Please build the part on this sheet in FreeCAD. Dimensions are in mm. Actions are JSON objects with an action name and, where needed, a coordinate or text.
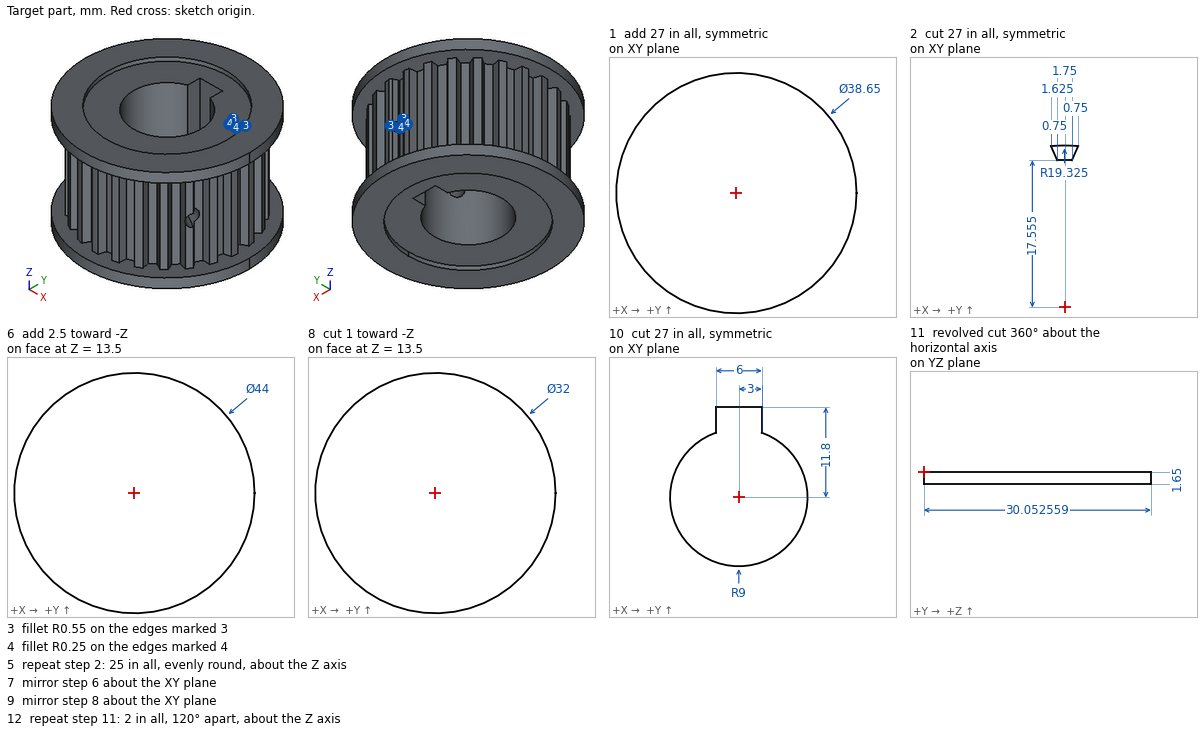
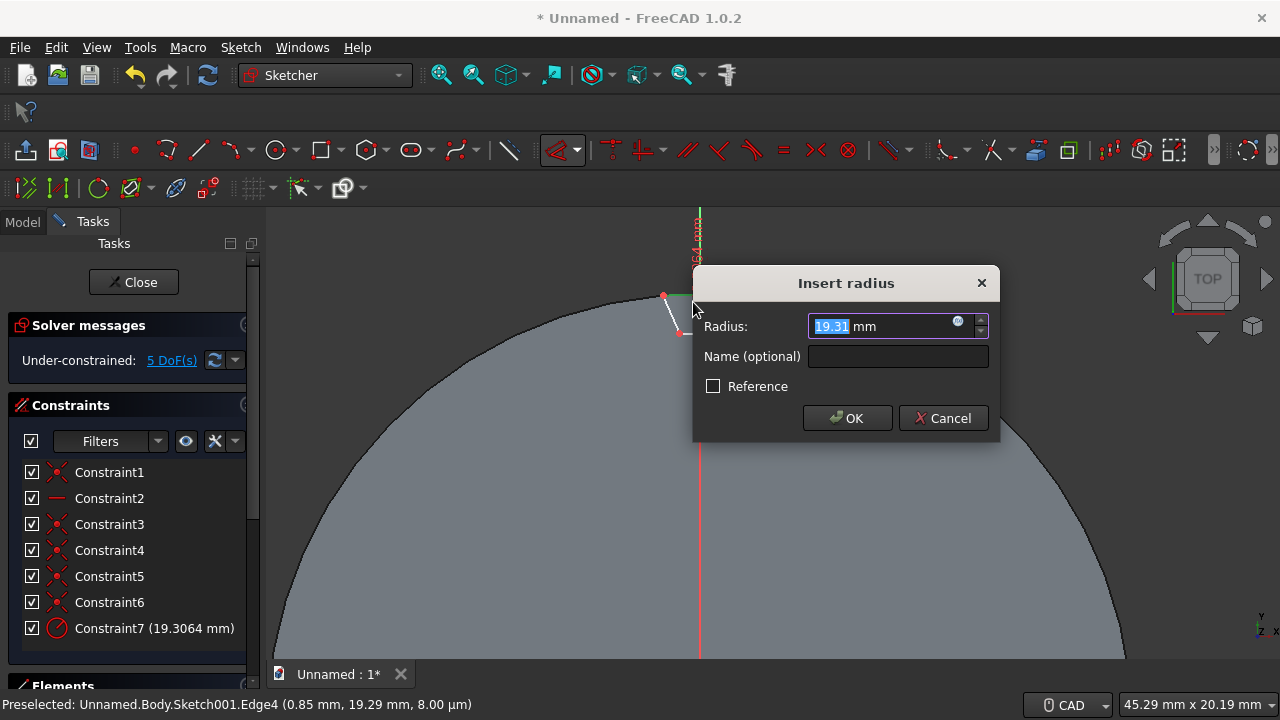
{"action": "type", "text": "19.325"}
{"action": "key", "text": "Return"}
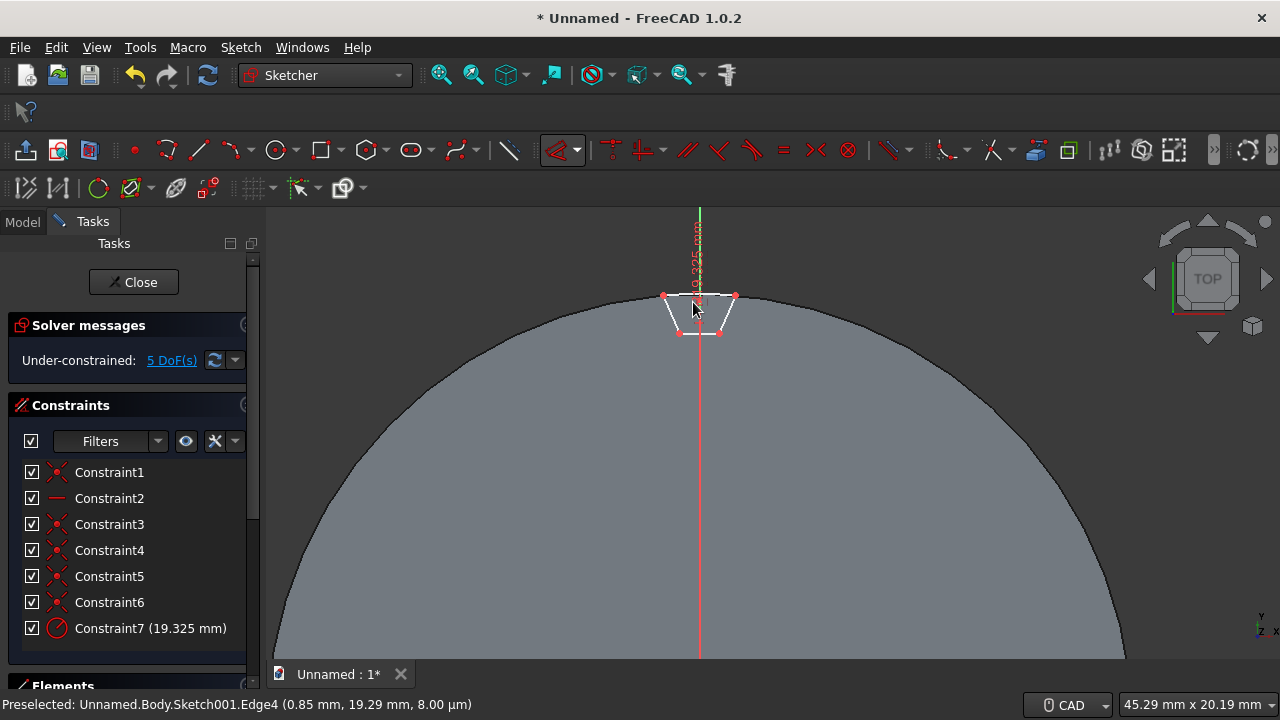
{"action": "left_click", "coordinate": [696, 334]}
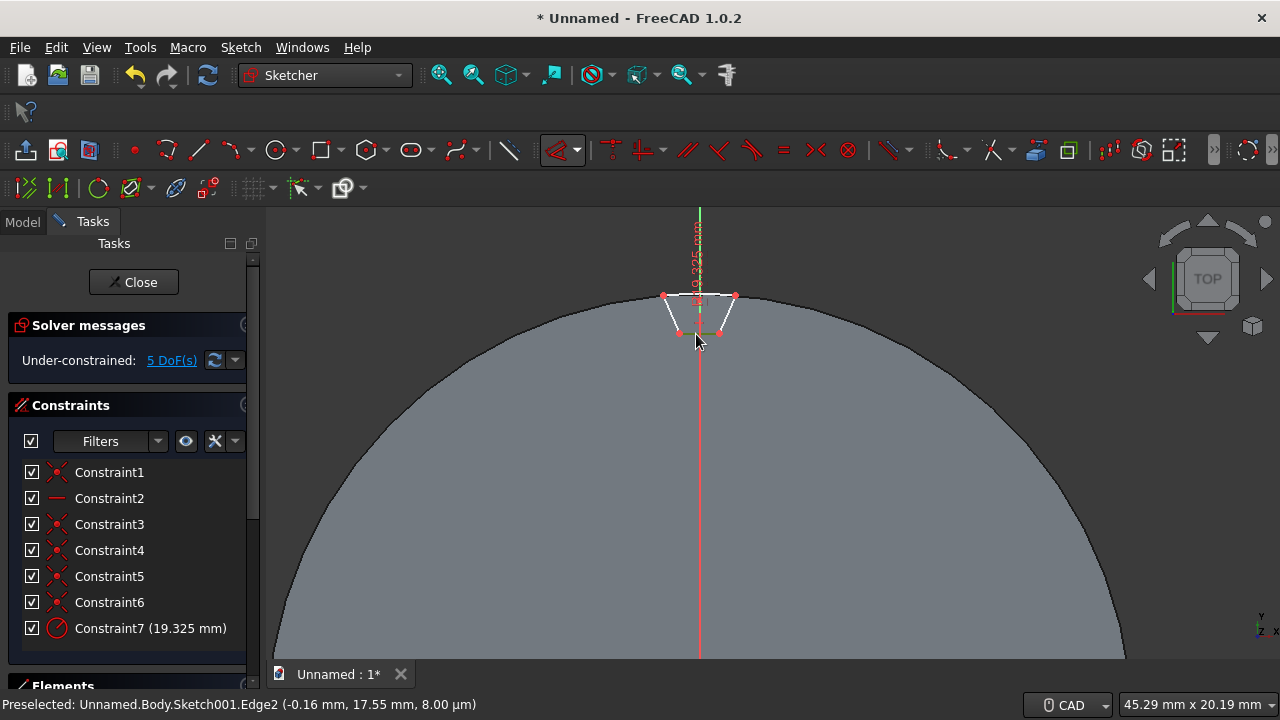
{"action": "key", "text": "l"}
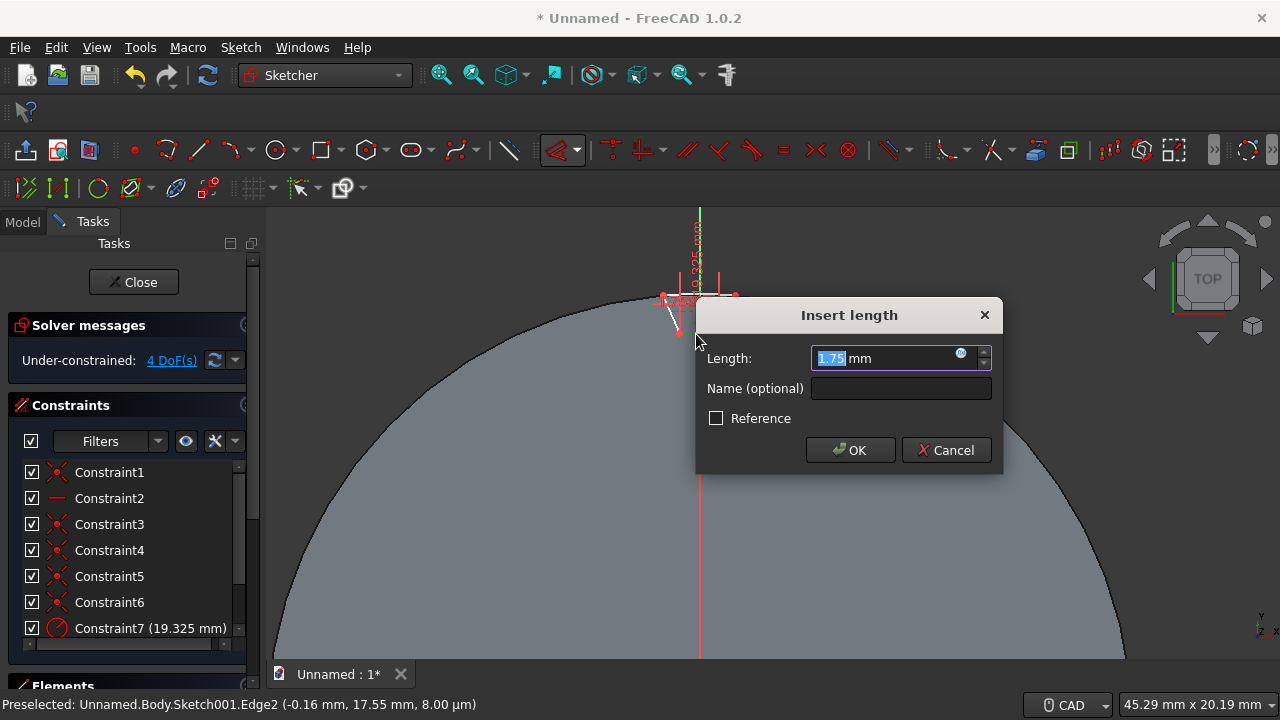
{"action": "type", "text": "1.75"}
{"action": "key", "text": "Return"}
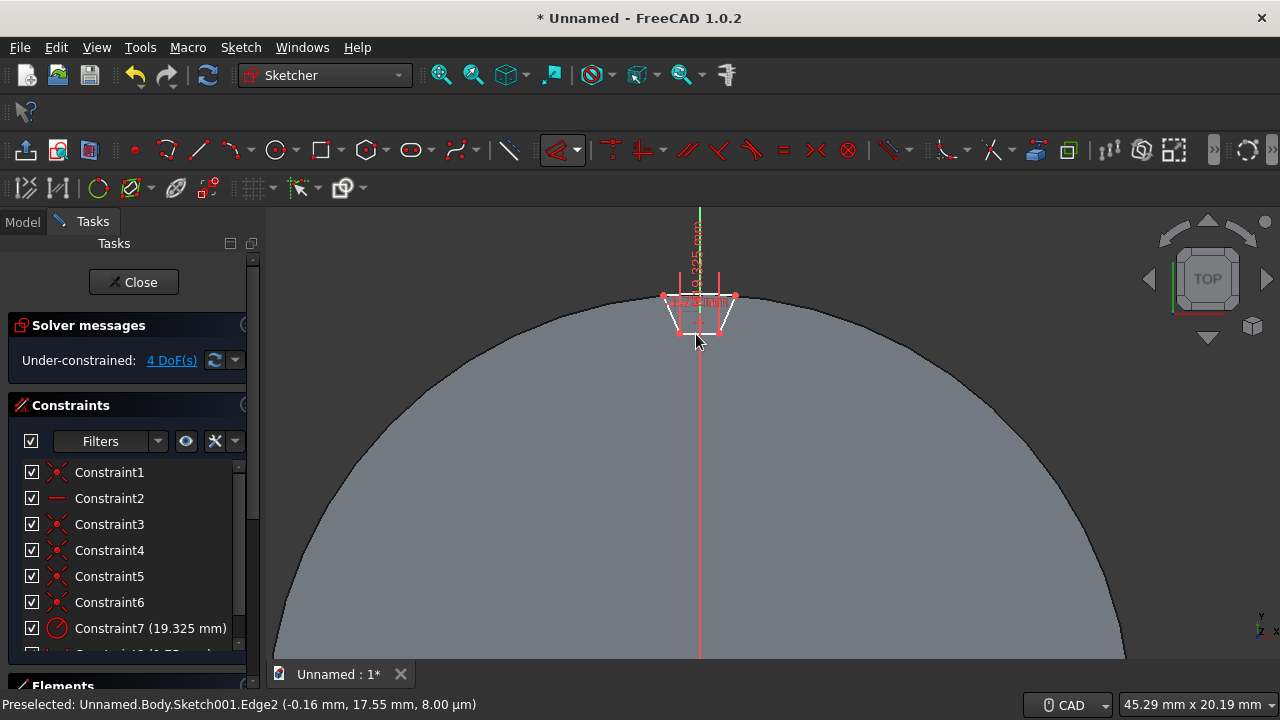
{"action": "scroll", "coordinate": [668, 307], "scroll_direction": "up", "scroll_amount": 5}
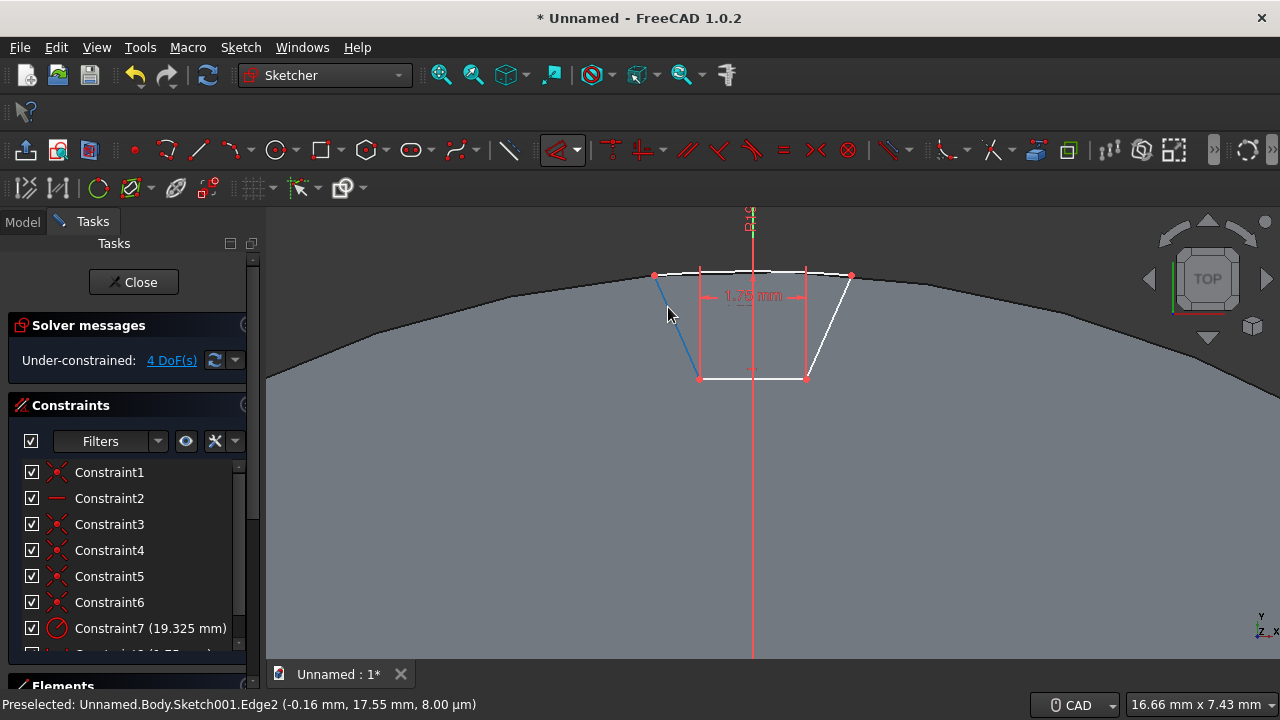
{"action": "left_click", "coordinate": [668, 307]}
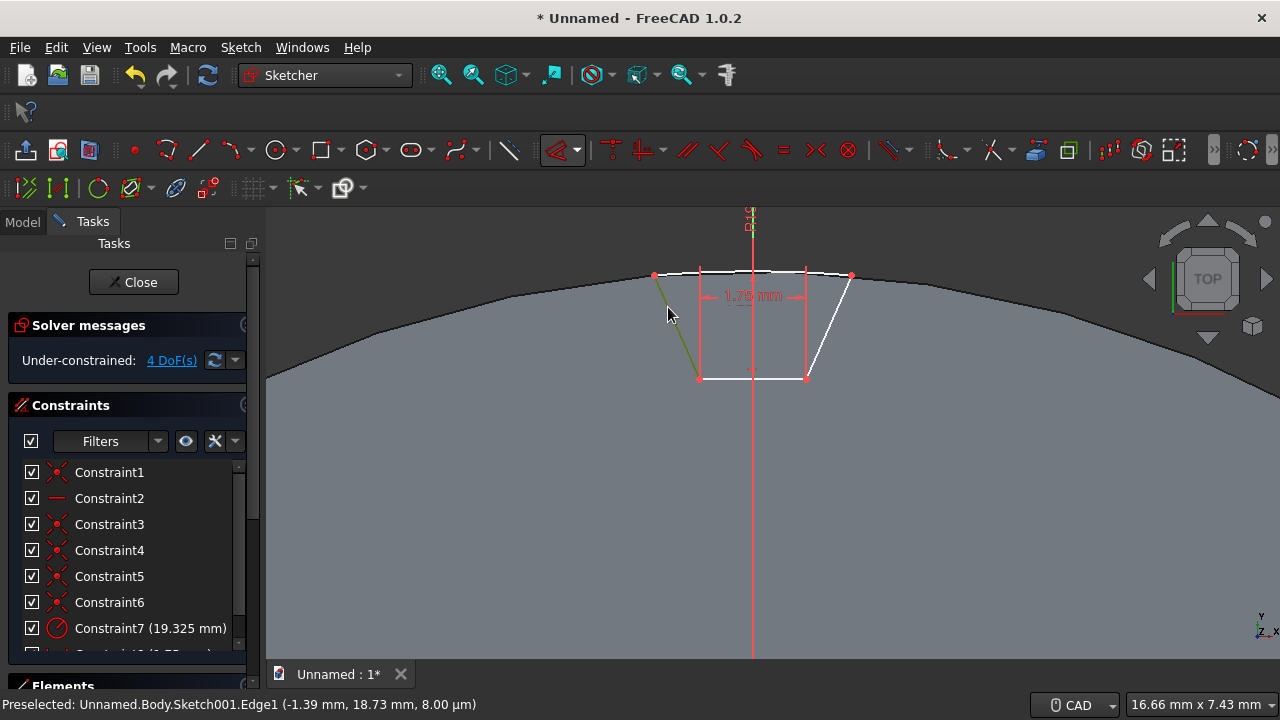
{"action": "key", "text": "l"}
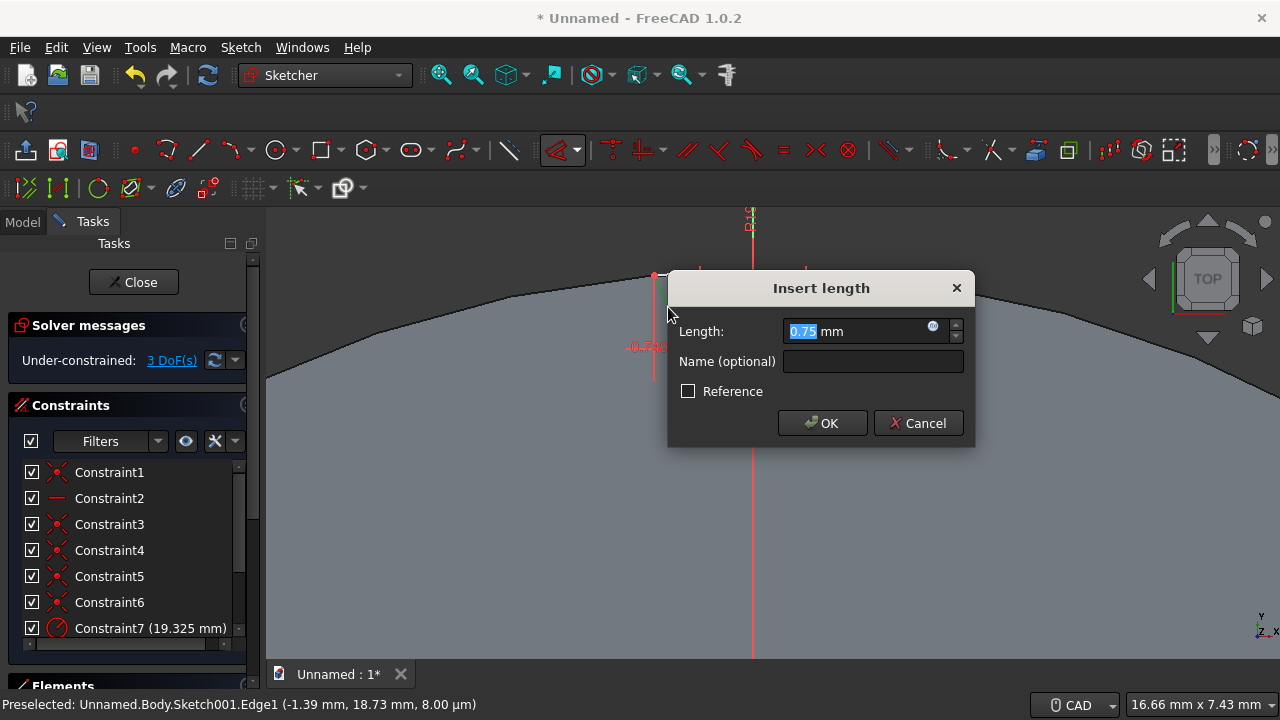
{"action": "type", "text": "0.75"}
{"action": "key", "text": "Return"}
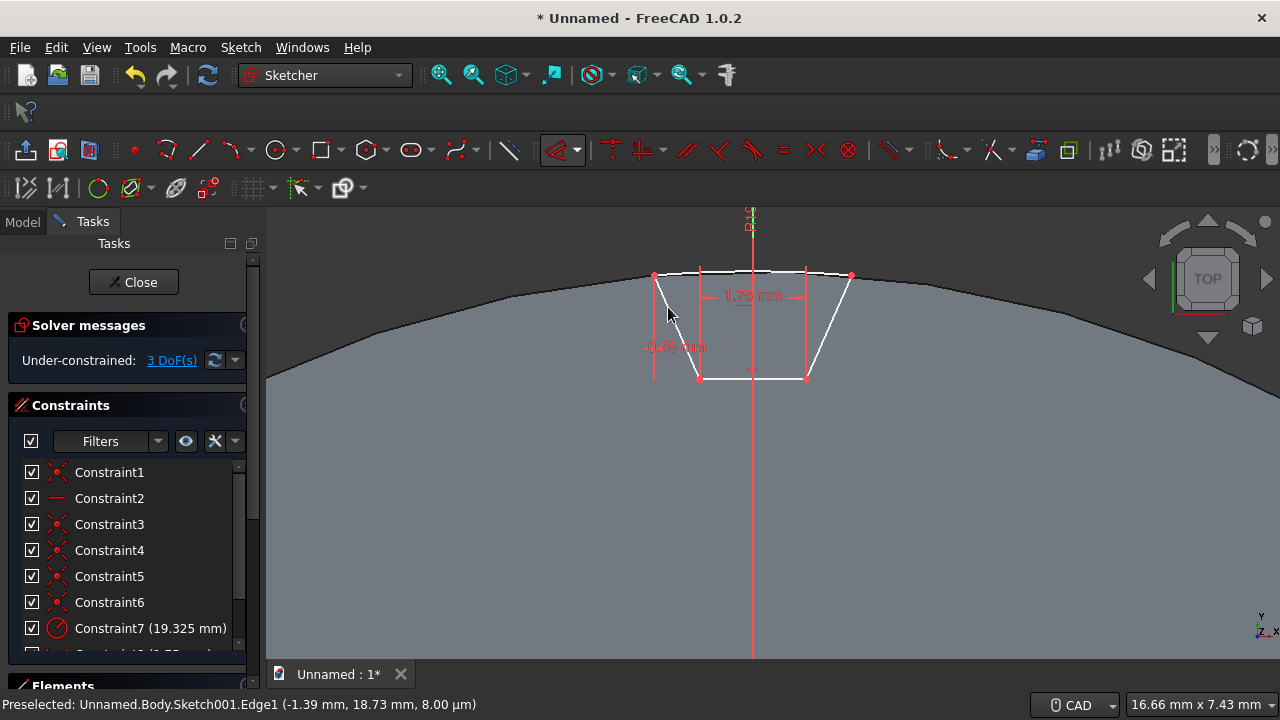
{"action": "left_click", "coordinate": [820, 348]}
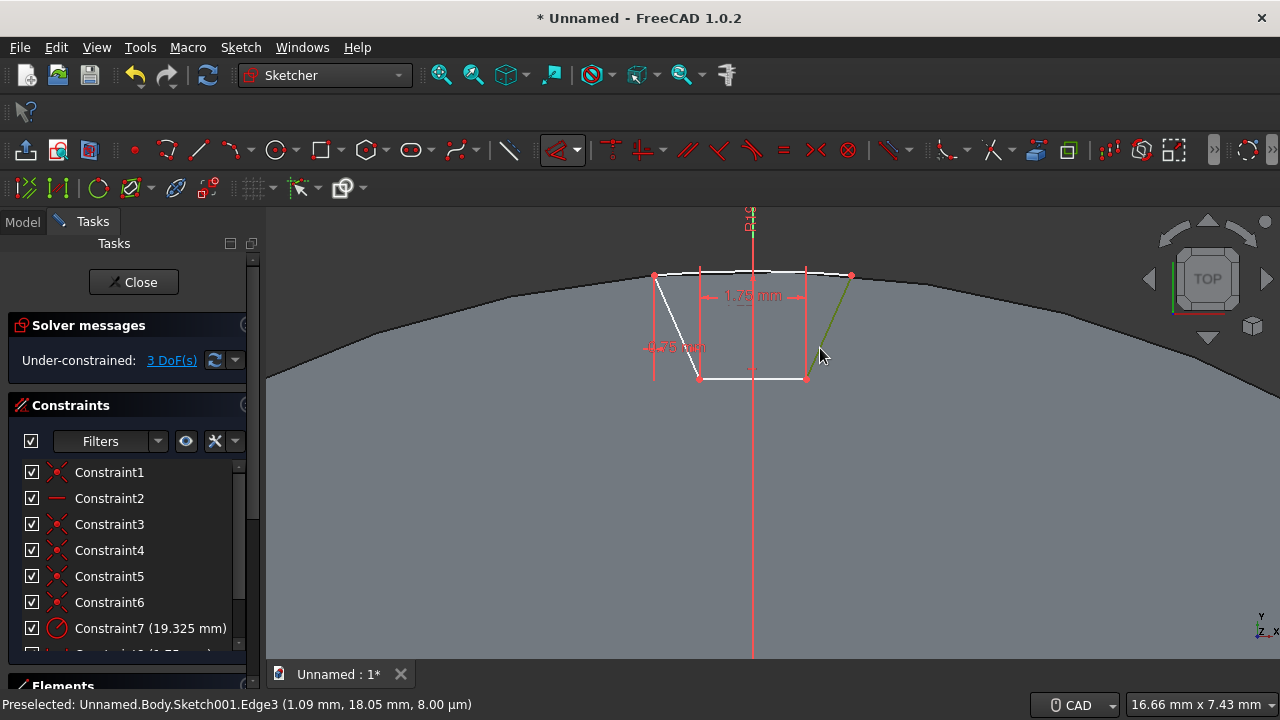
{"action": "key", "text": "l"}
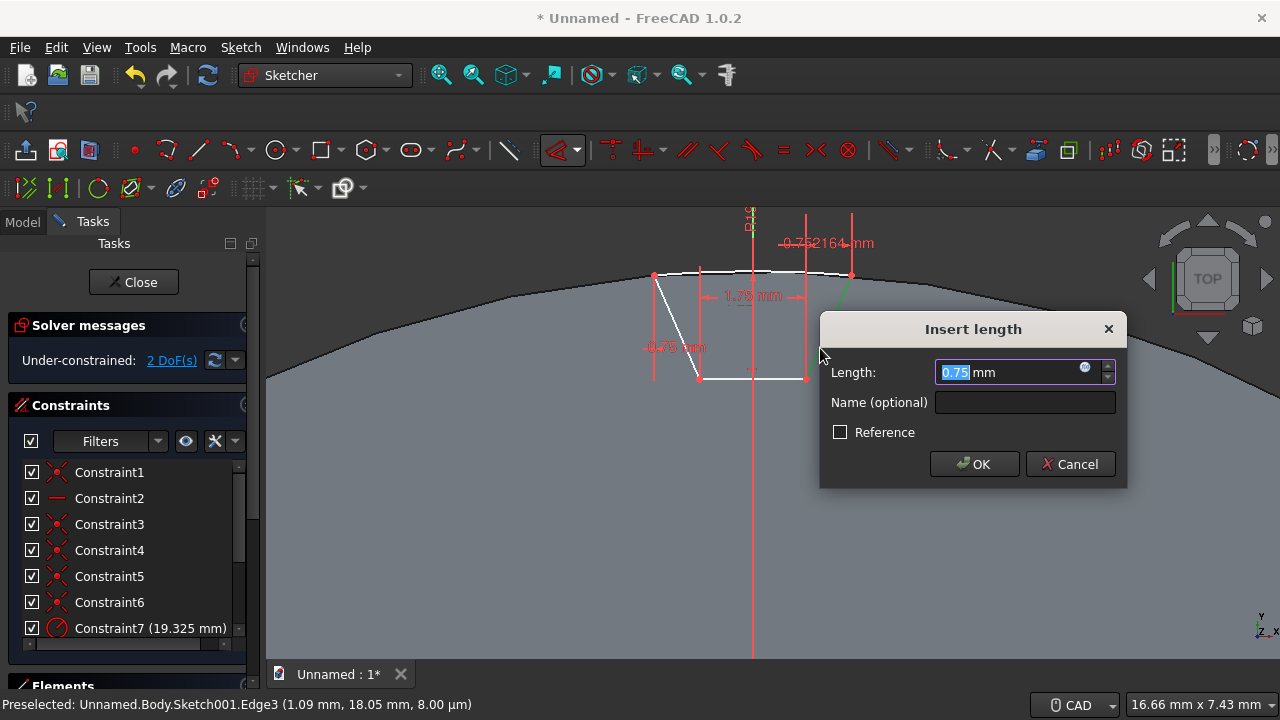
{"action": "type", "text": "0.75"}
{"action": "key", "text": "Return"}